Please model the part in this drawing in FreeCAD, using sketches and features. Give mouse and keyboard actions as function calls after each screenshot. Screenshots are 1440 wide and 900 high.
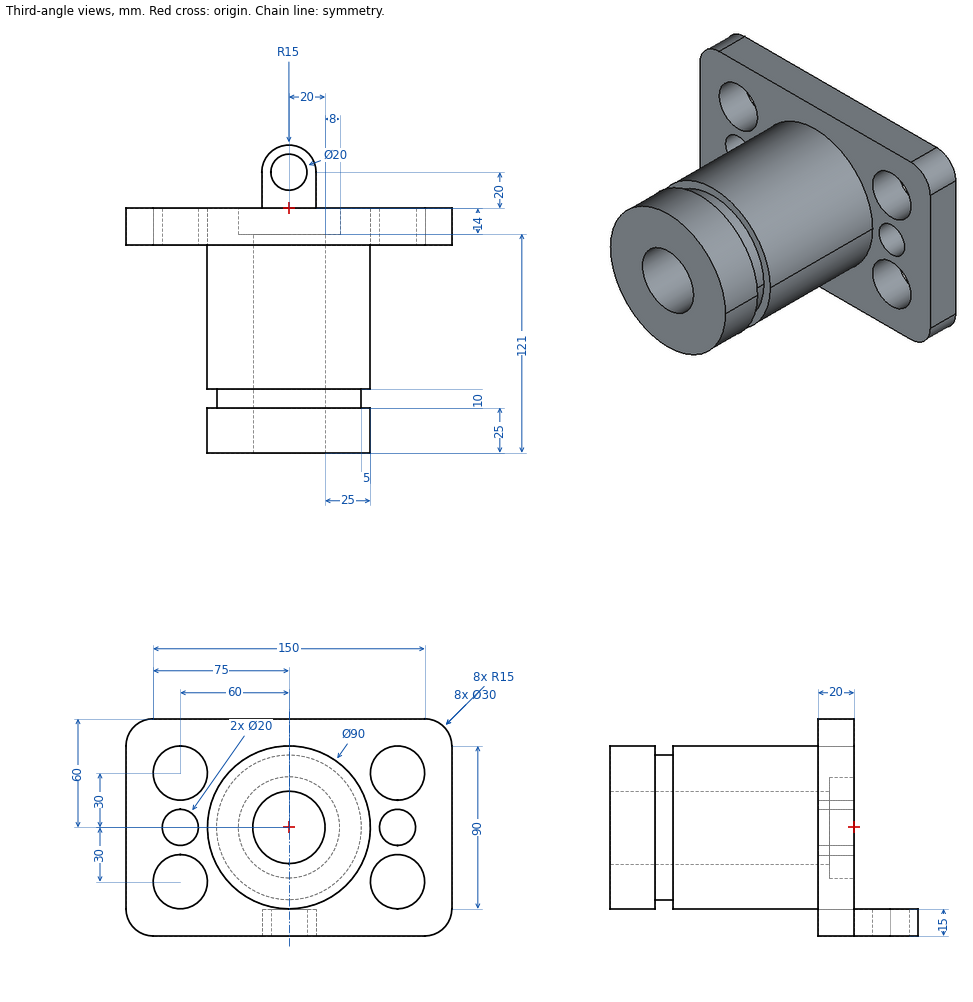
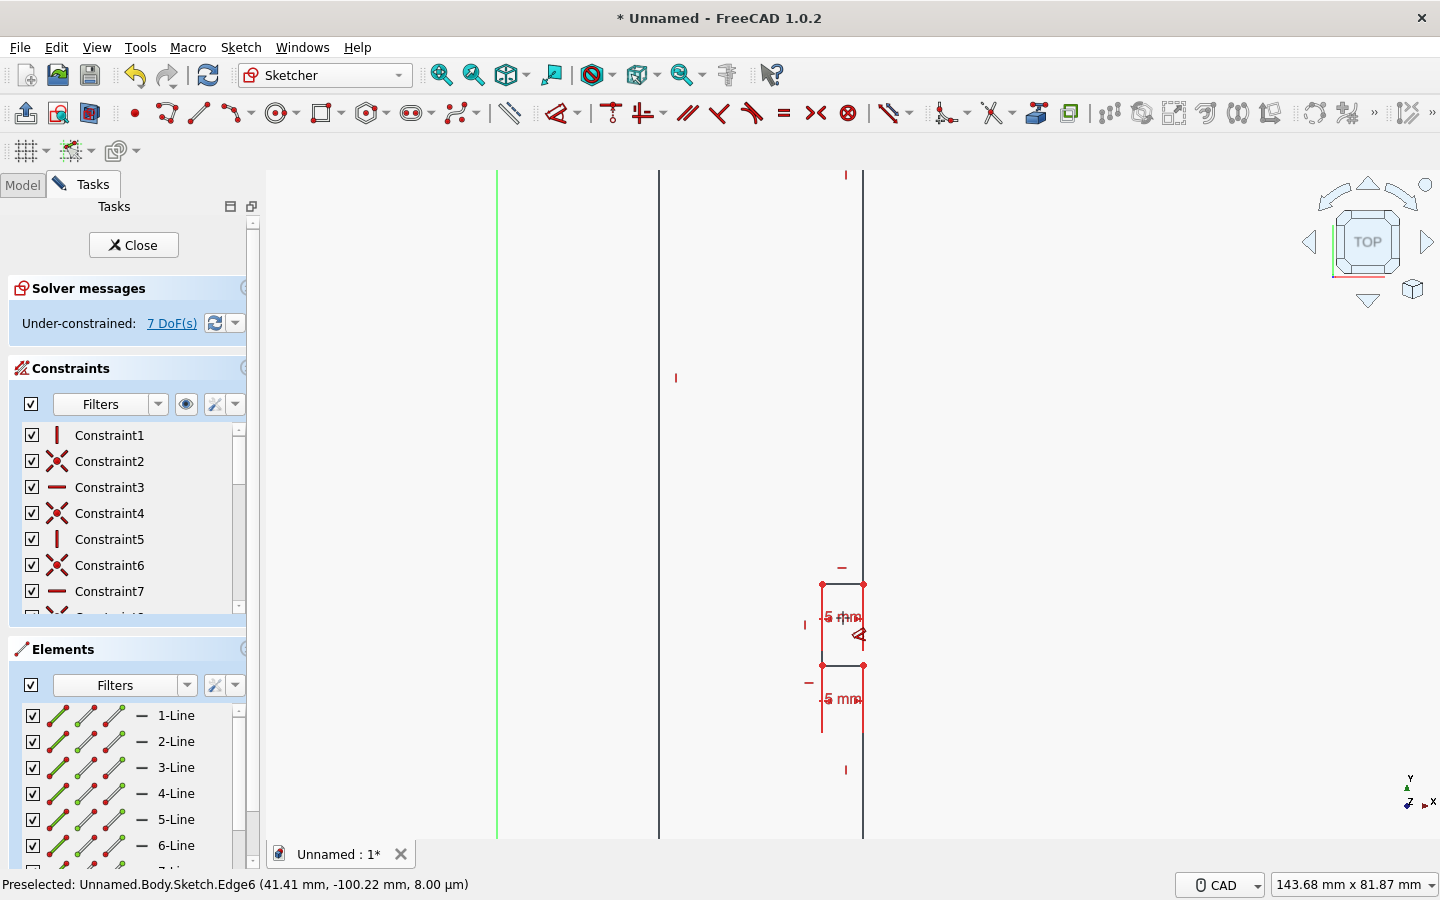
scroll(845, 614, down, 5)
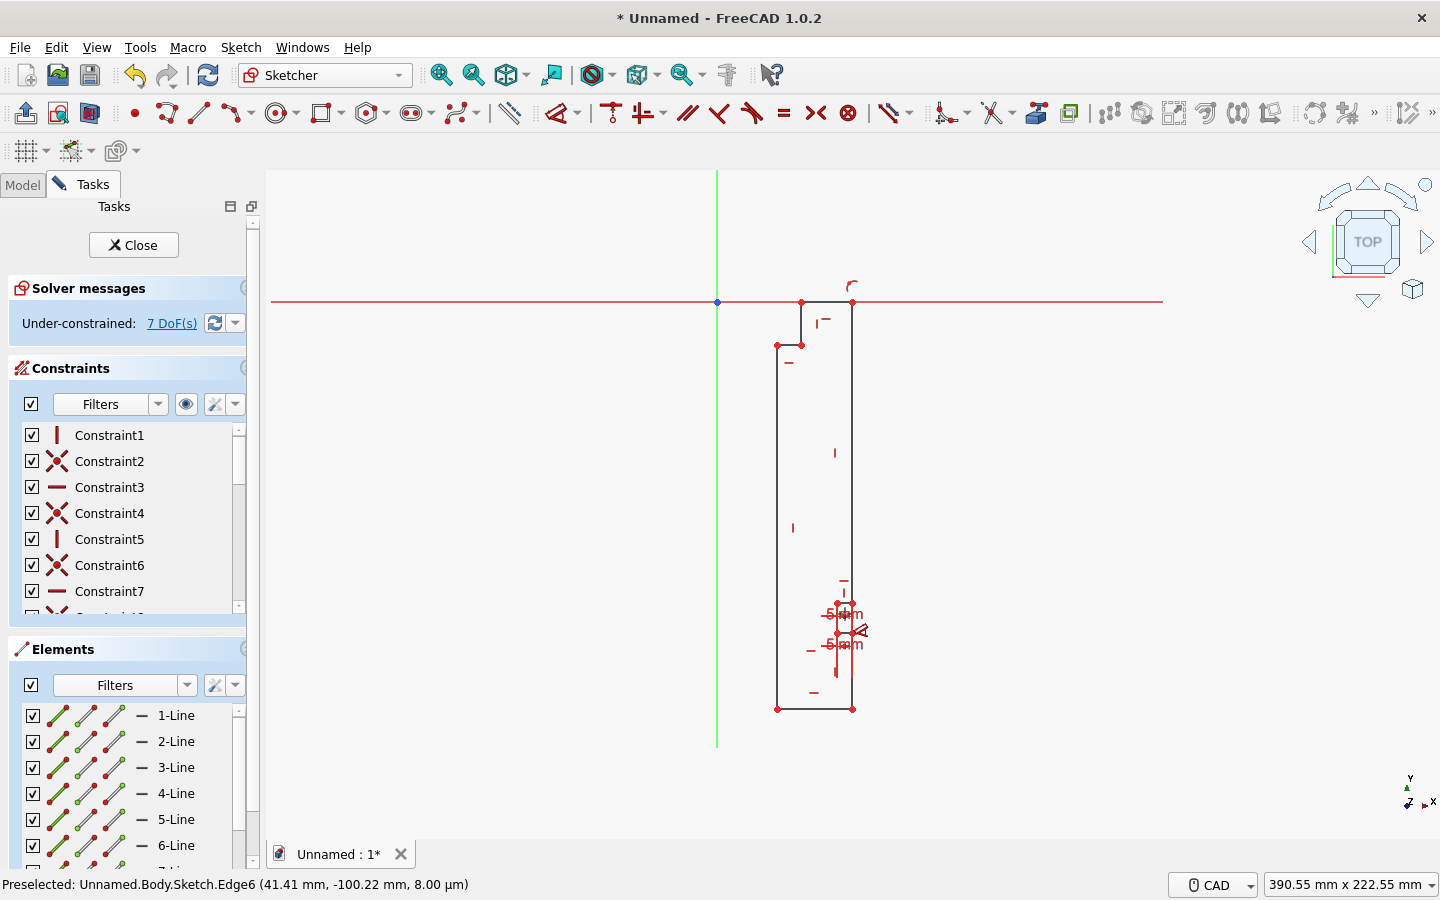
scroll(794, 345, up, 4)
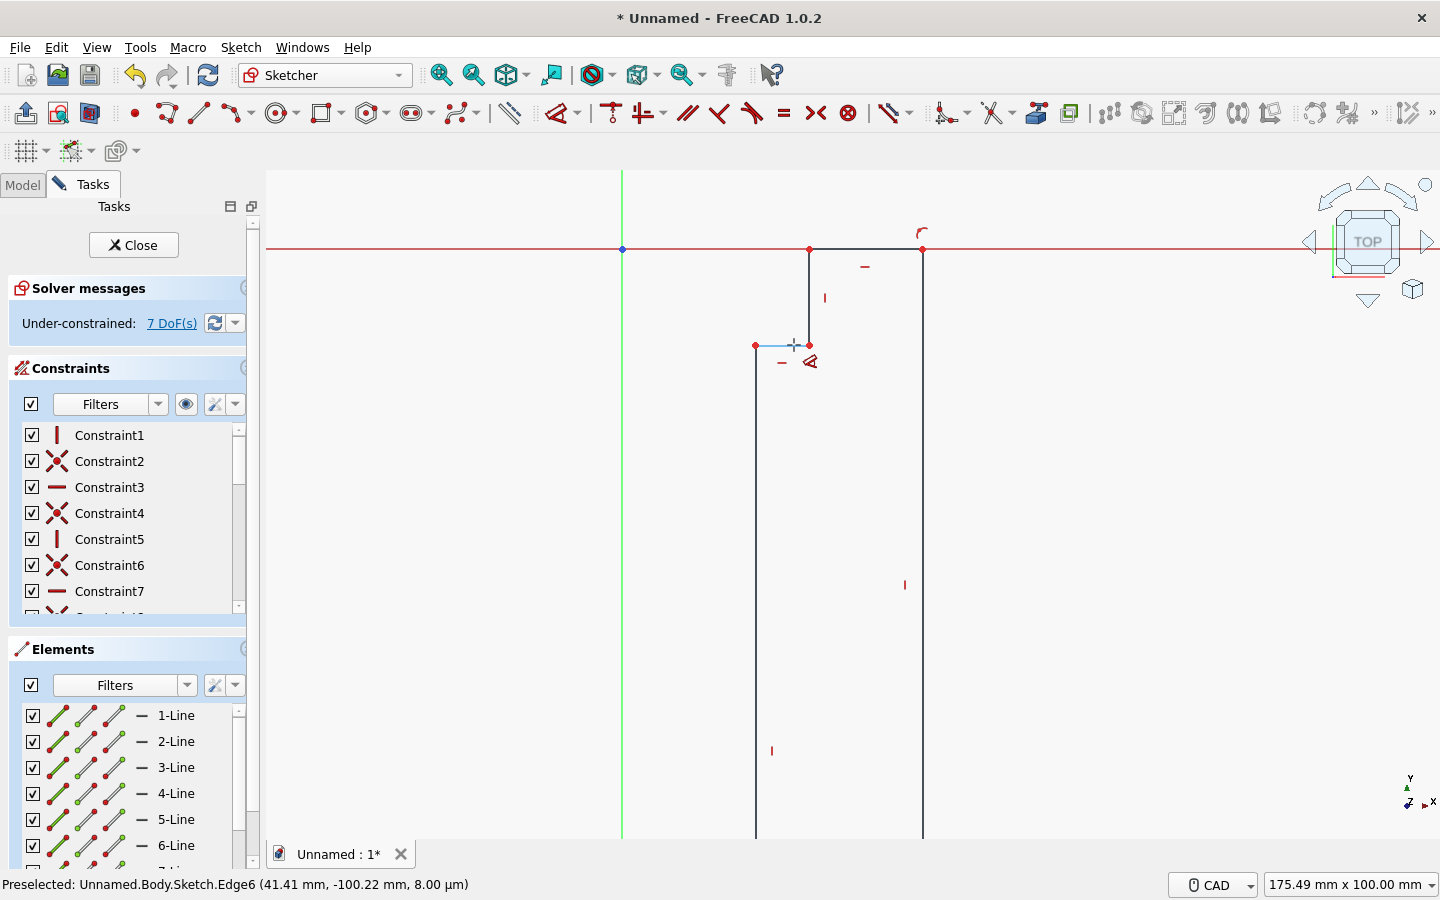
click(793, 346)
click(782, 312)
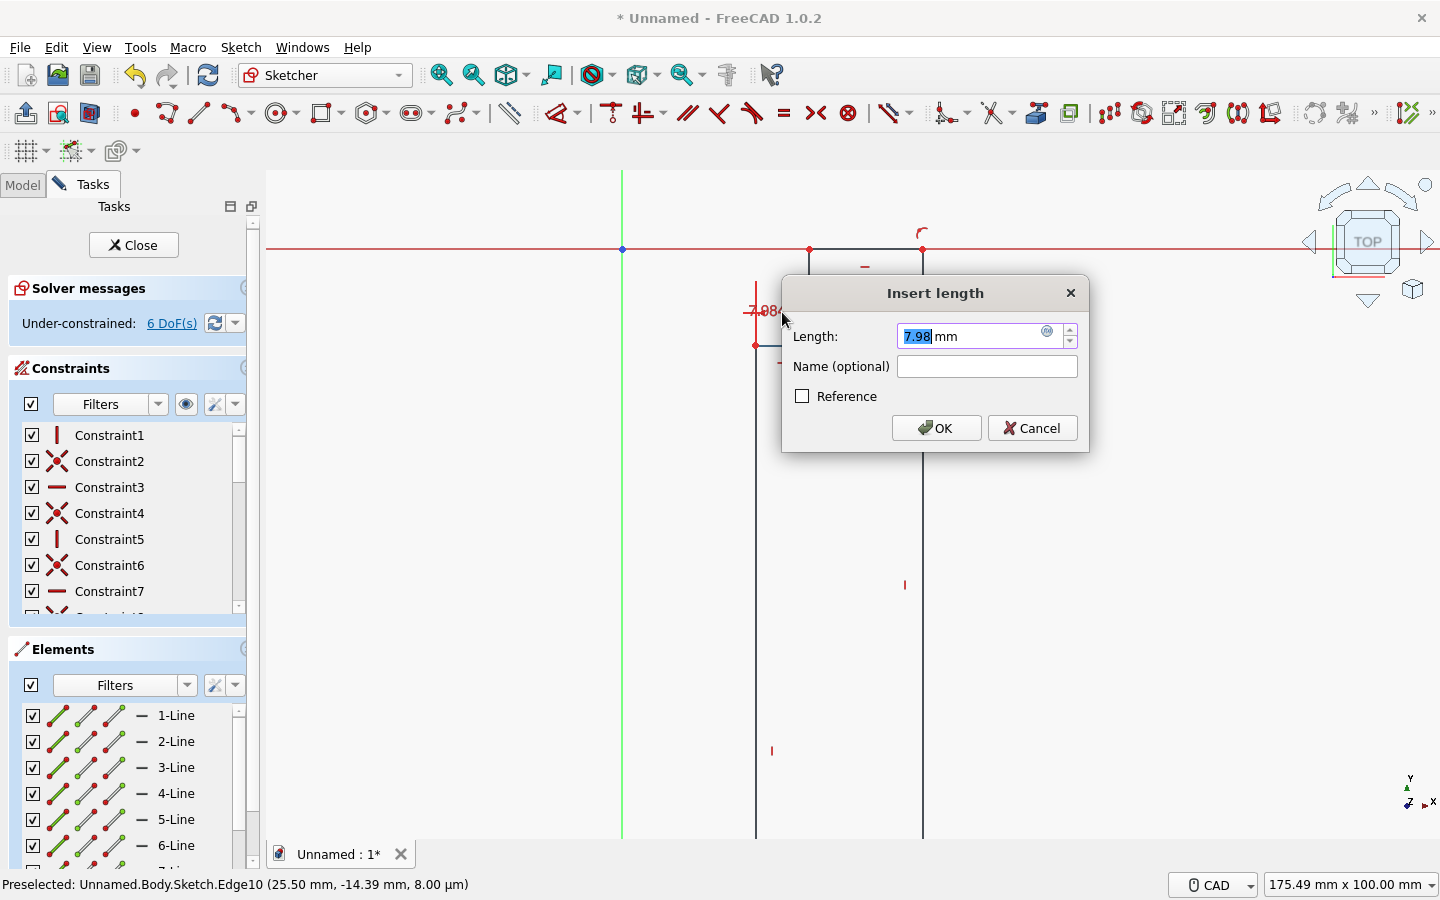
text(8)
key(Return)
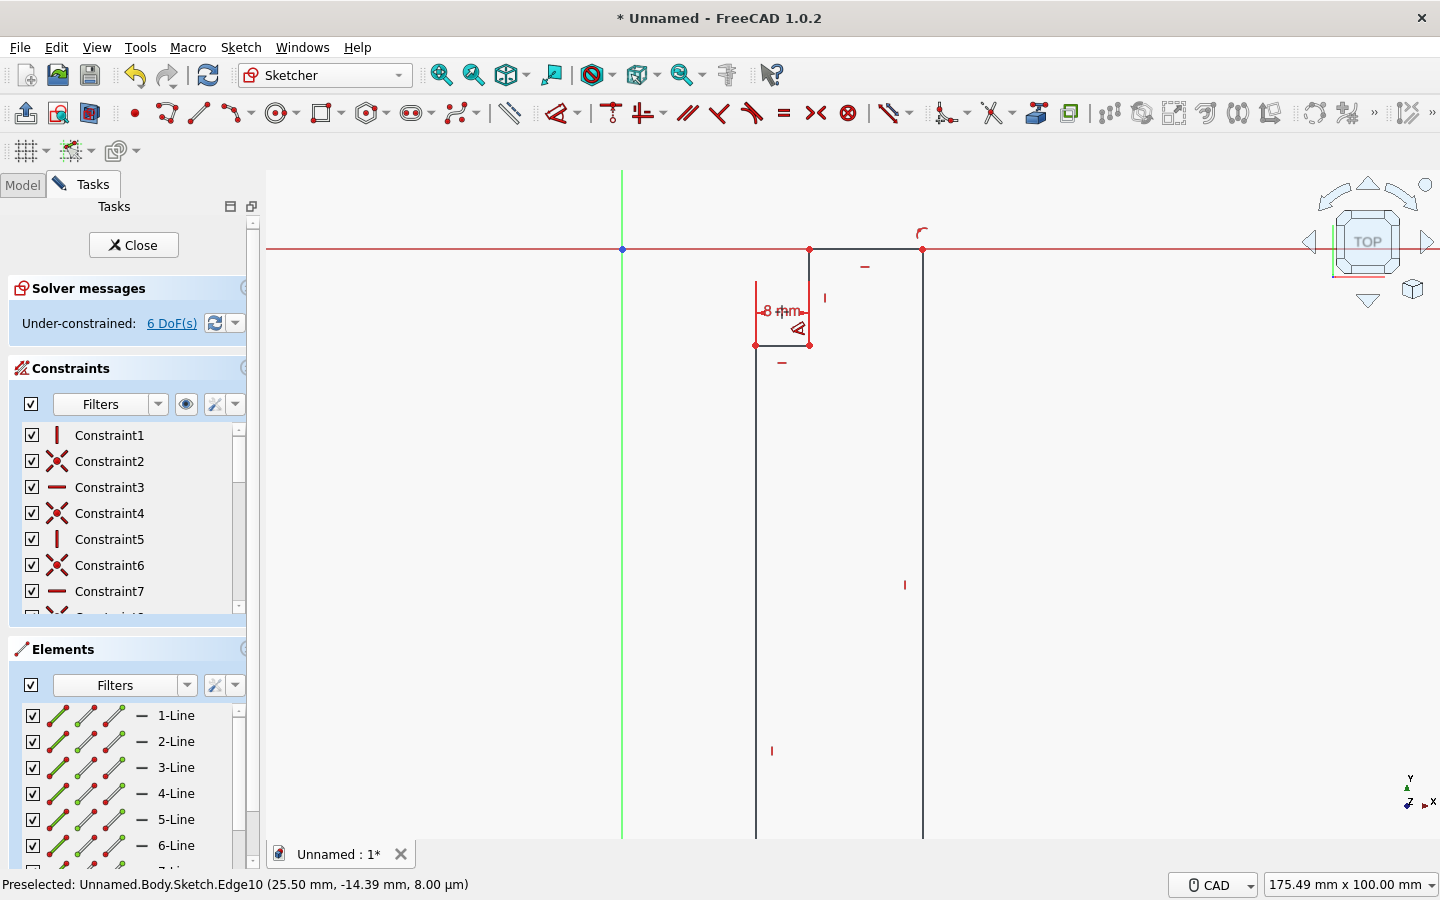
scroll(794, 344, down, 4)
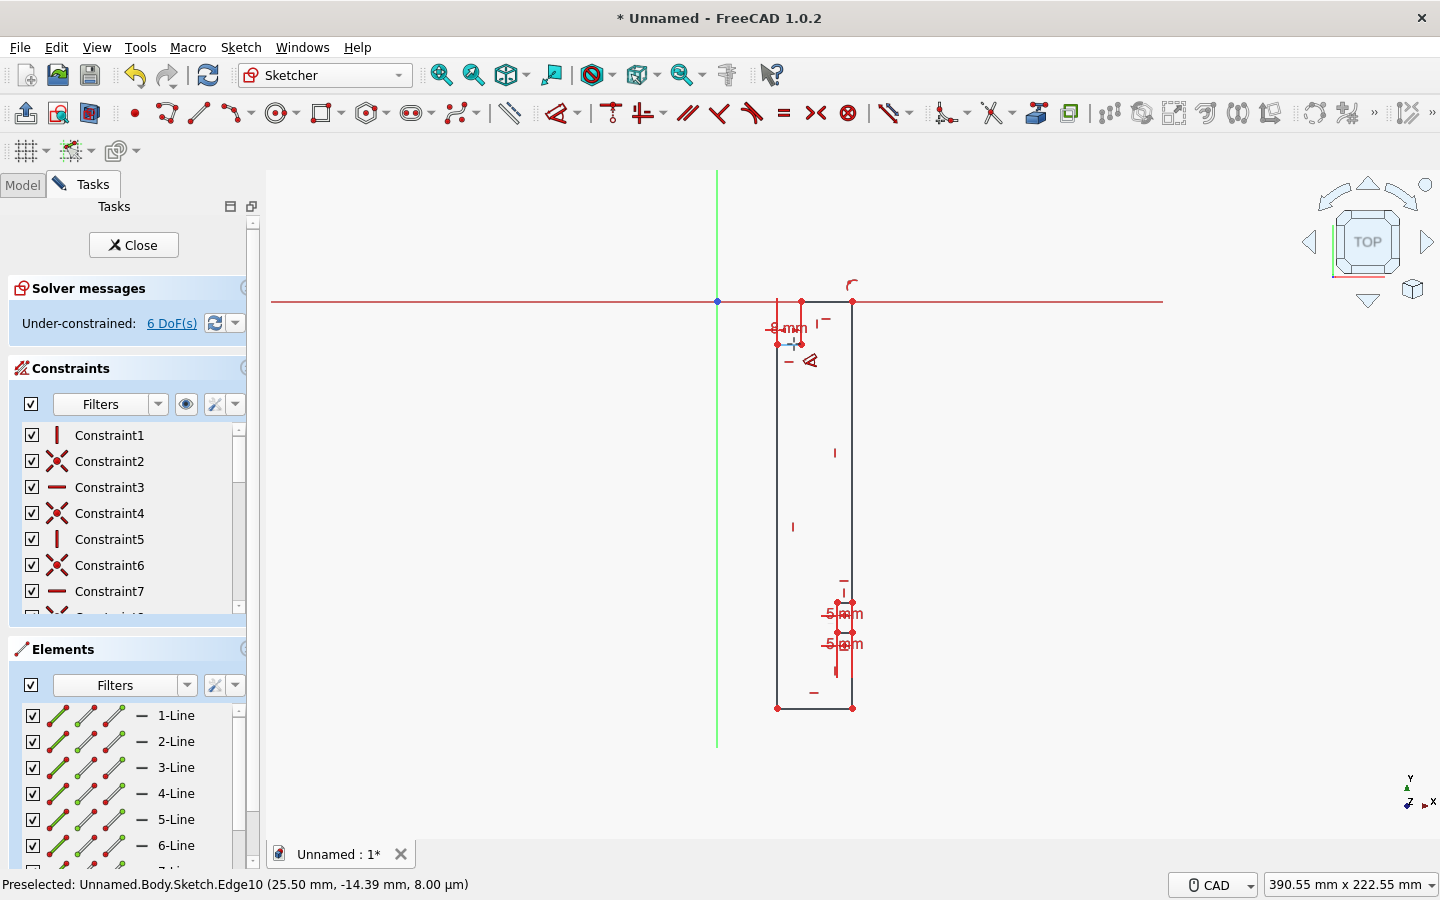
click(800, 709)
click(815, 743)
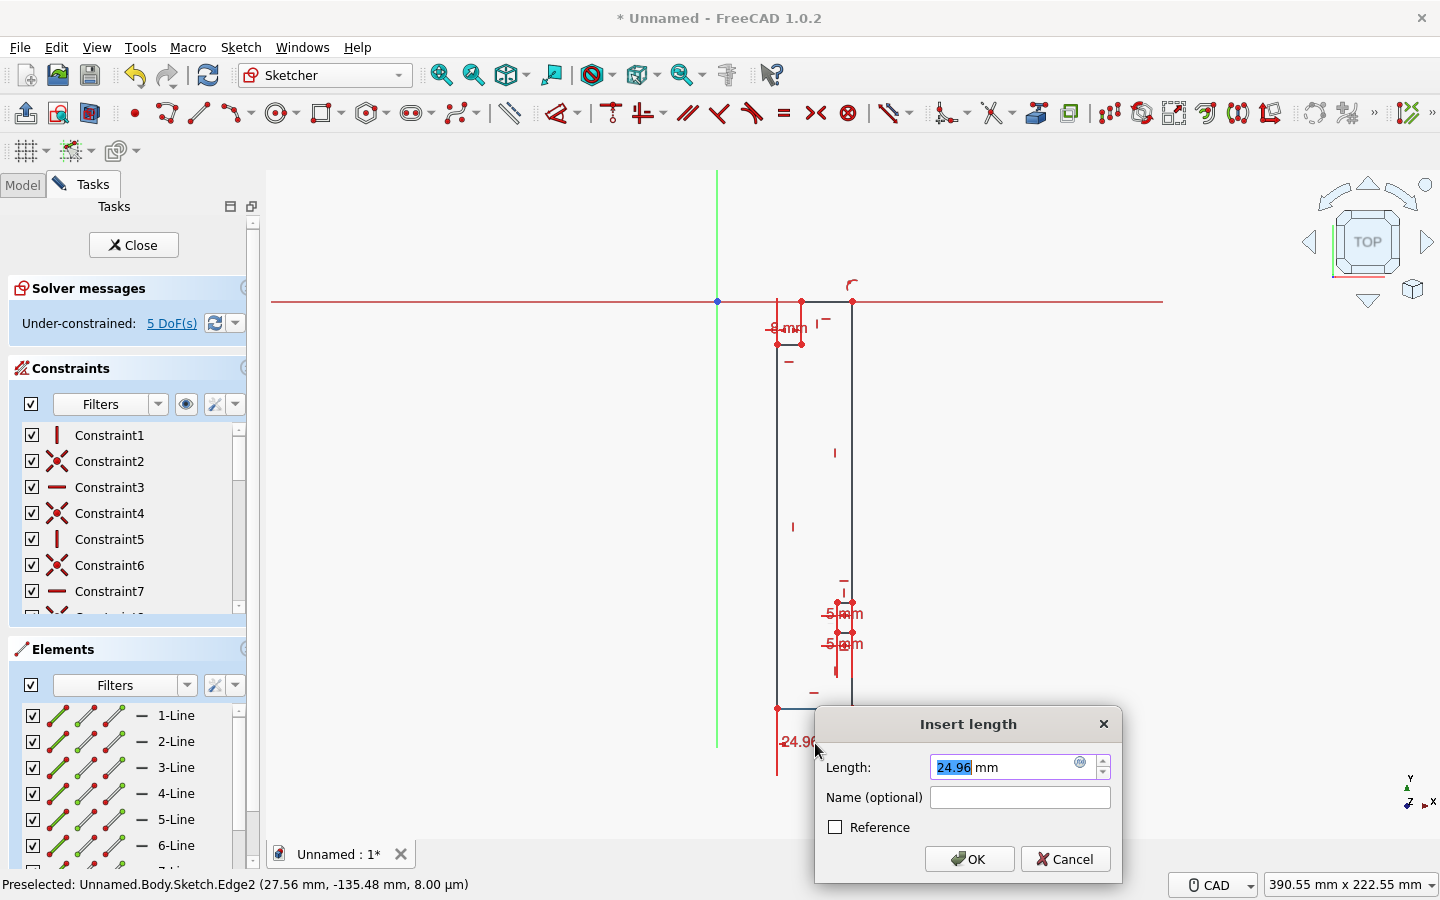
text(25)
key(Return)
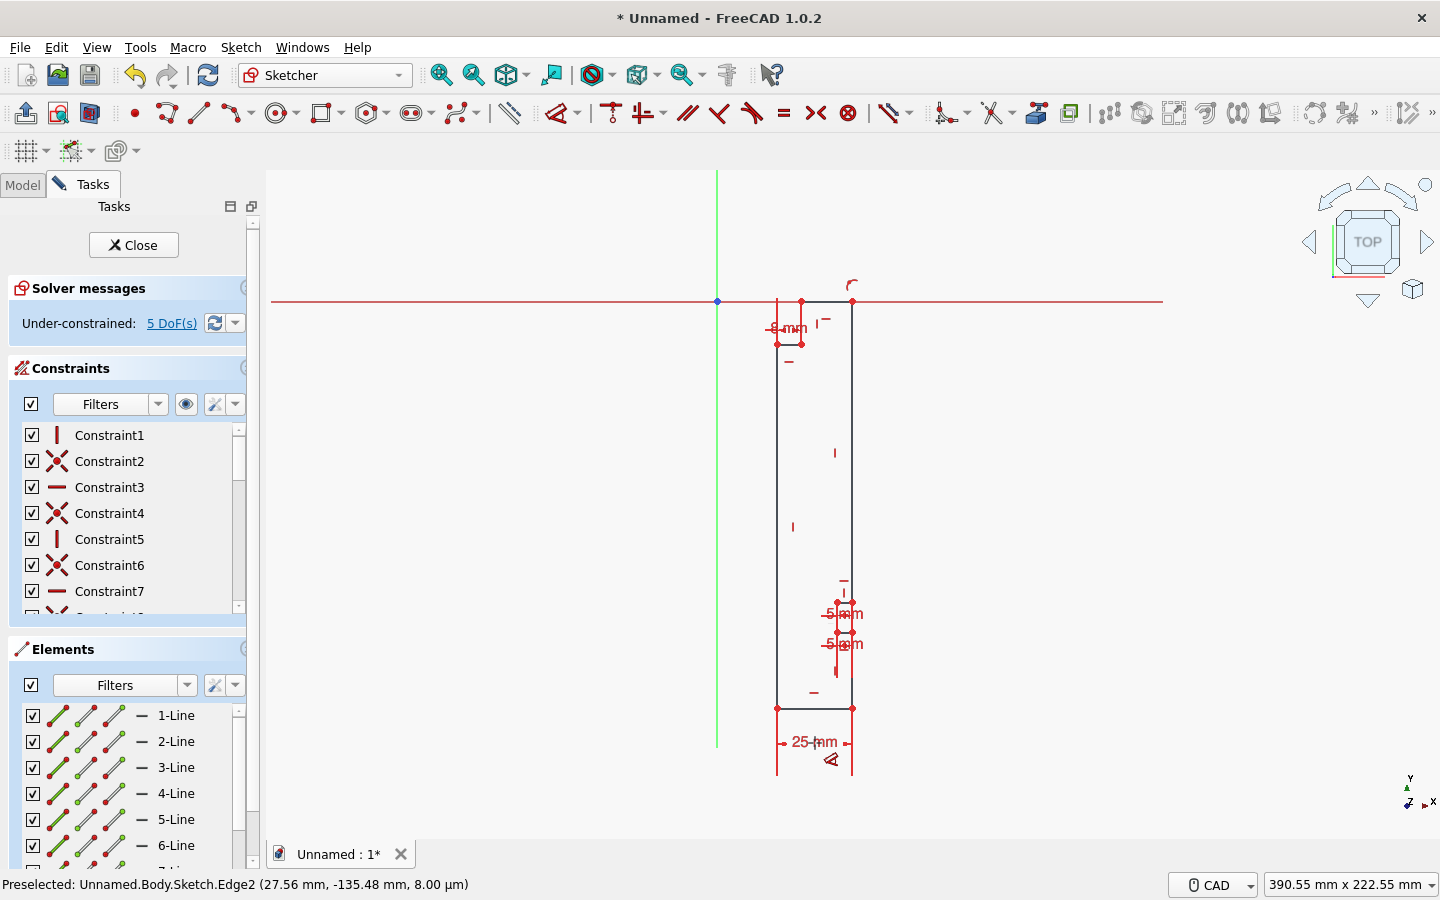
click(852, 686)
click(886, 671)